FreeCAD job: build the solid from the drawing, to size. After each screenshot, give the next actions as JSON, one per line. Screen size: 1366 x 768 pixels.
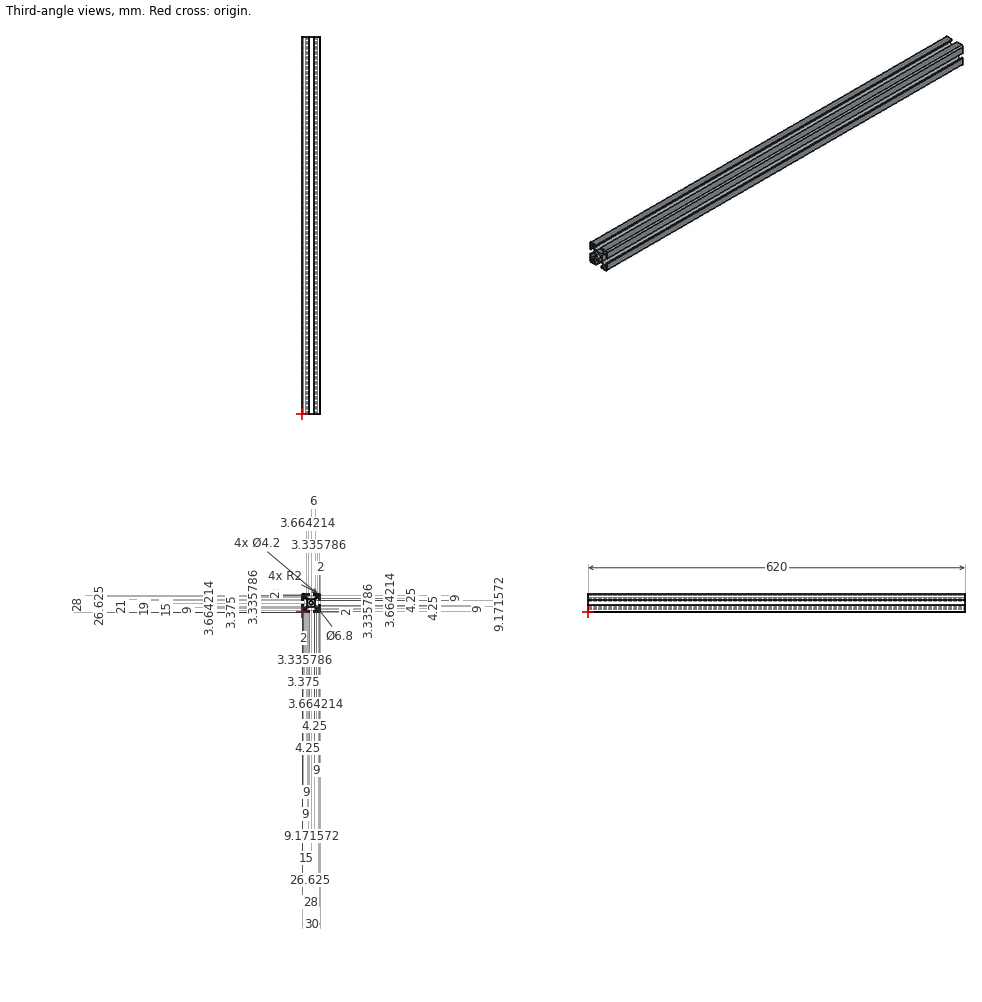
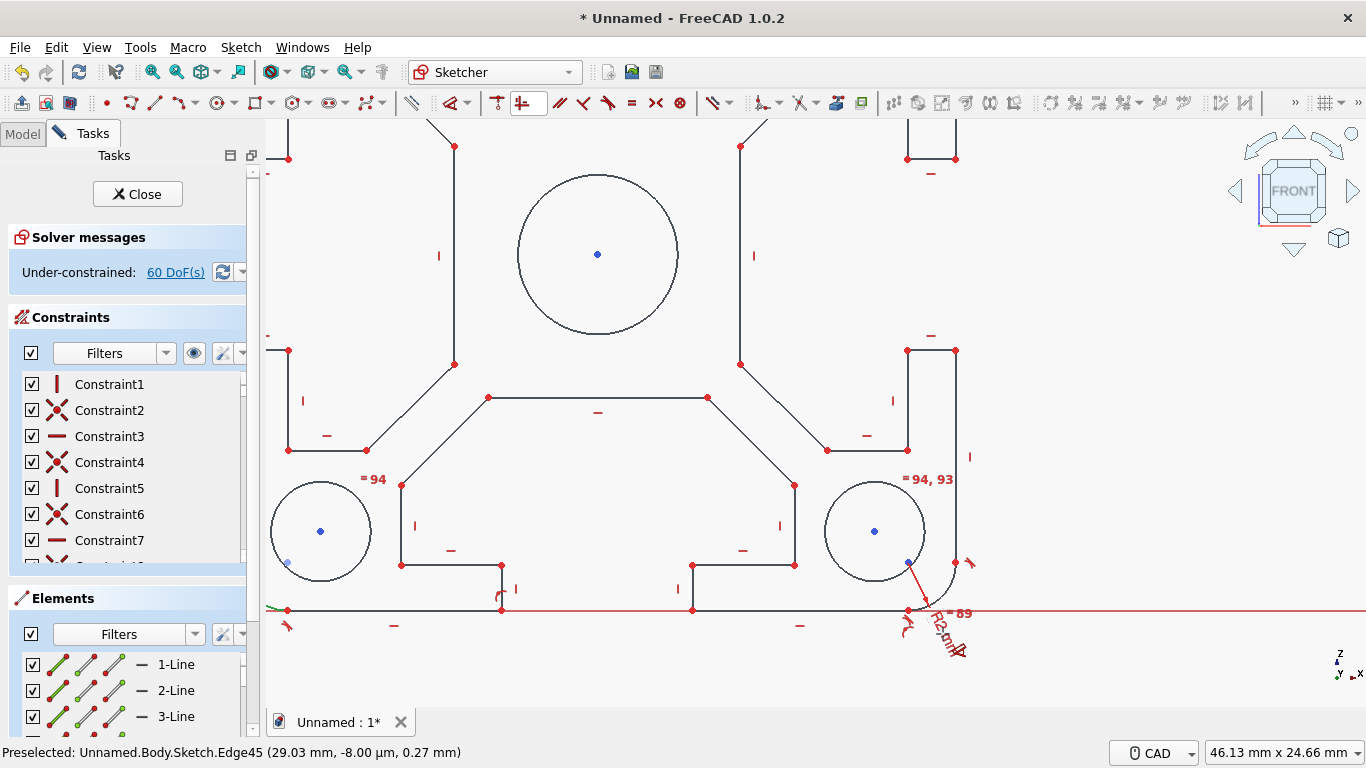
{"action": "scroll", "coordinate": [930, 608], "scroll_direction": "down", "scroll_amount": 3}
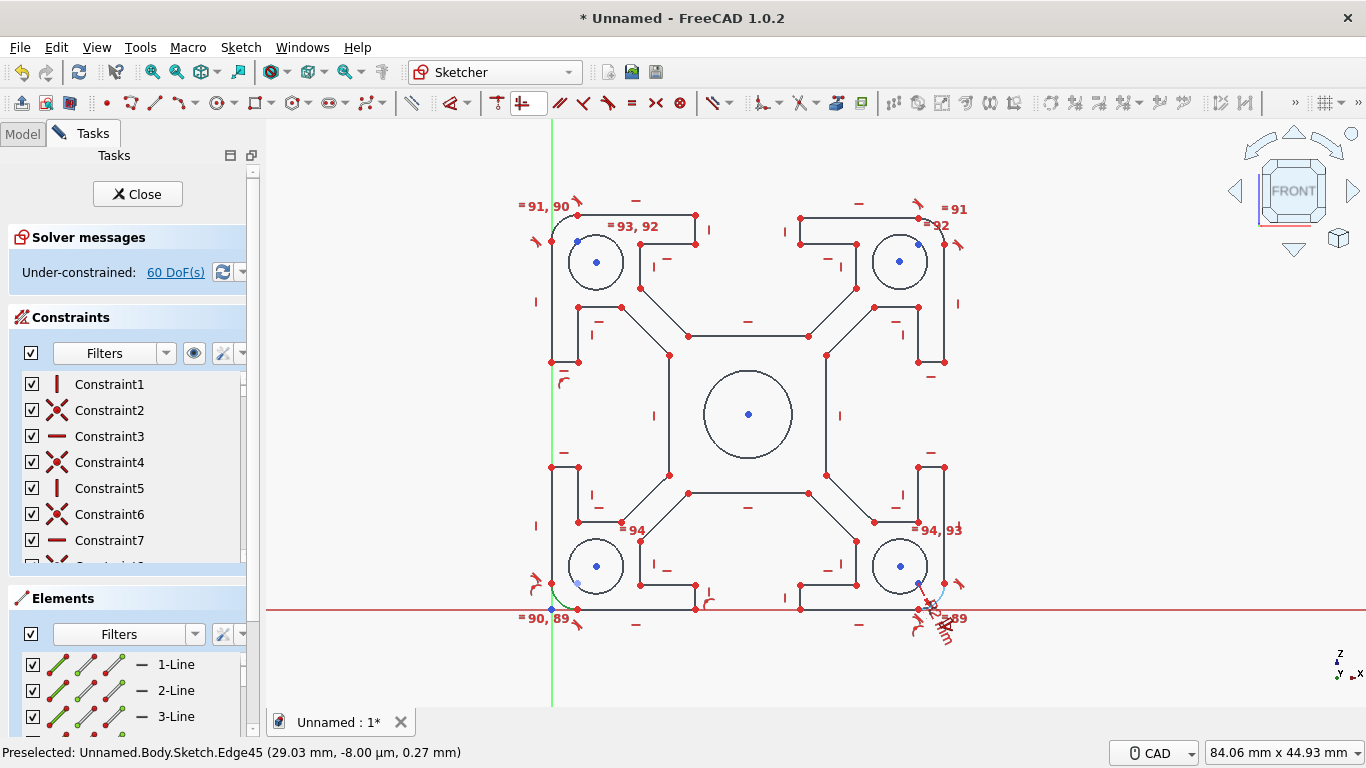
{"action": "left_click", "coordinate": [881, 243]}
{"action": "left_click", "coordinate": [912, 204]}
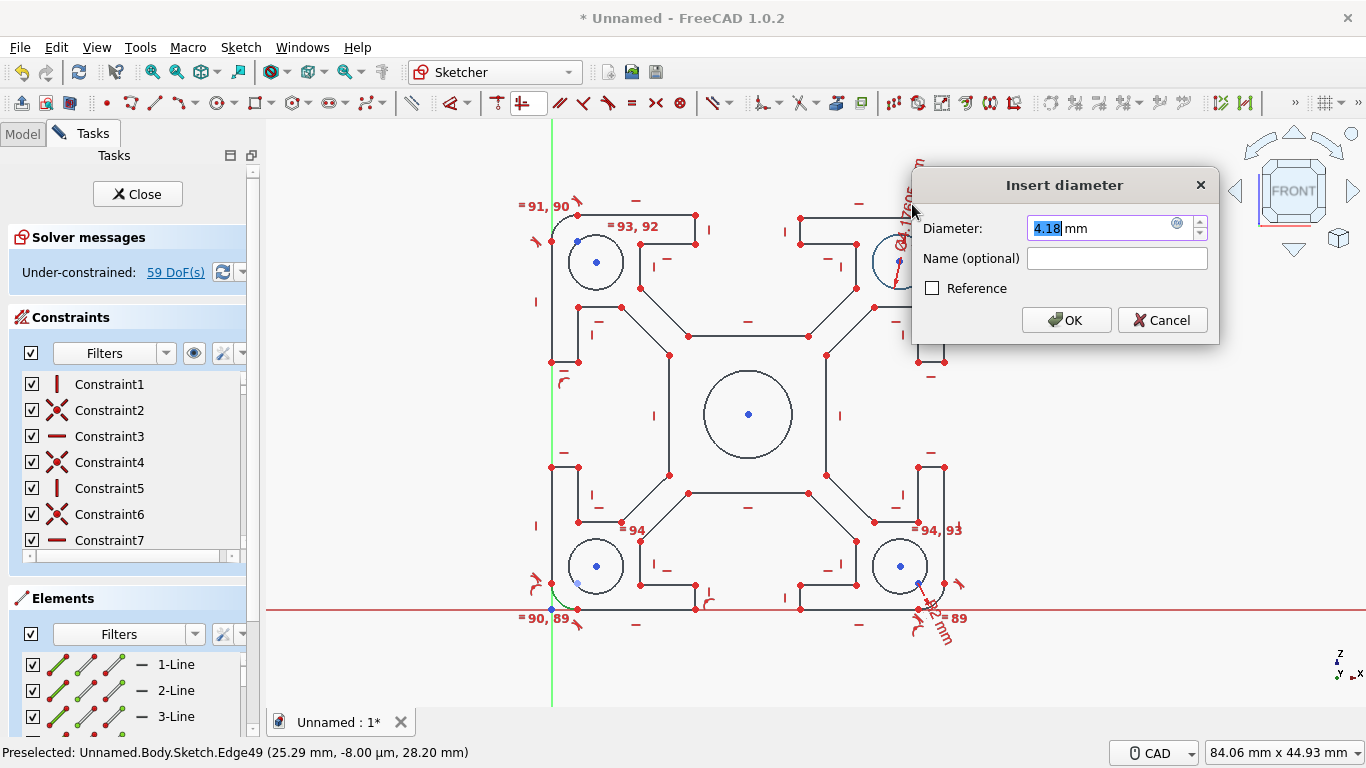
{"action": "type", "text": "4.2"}
{"action": "key", "text": "Return"}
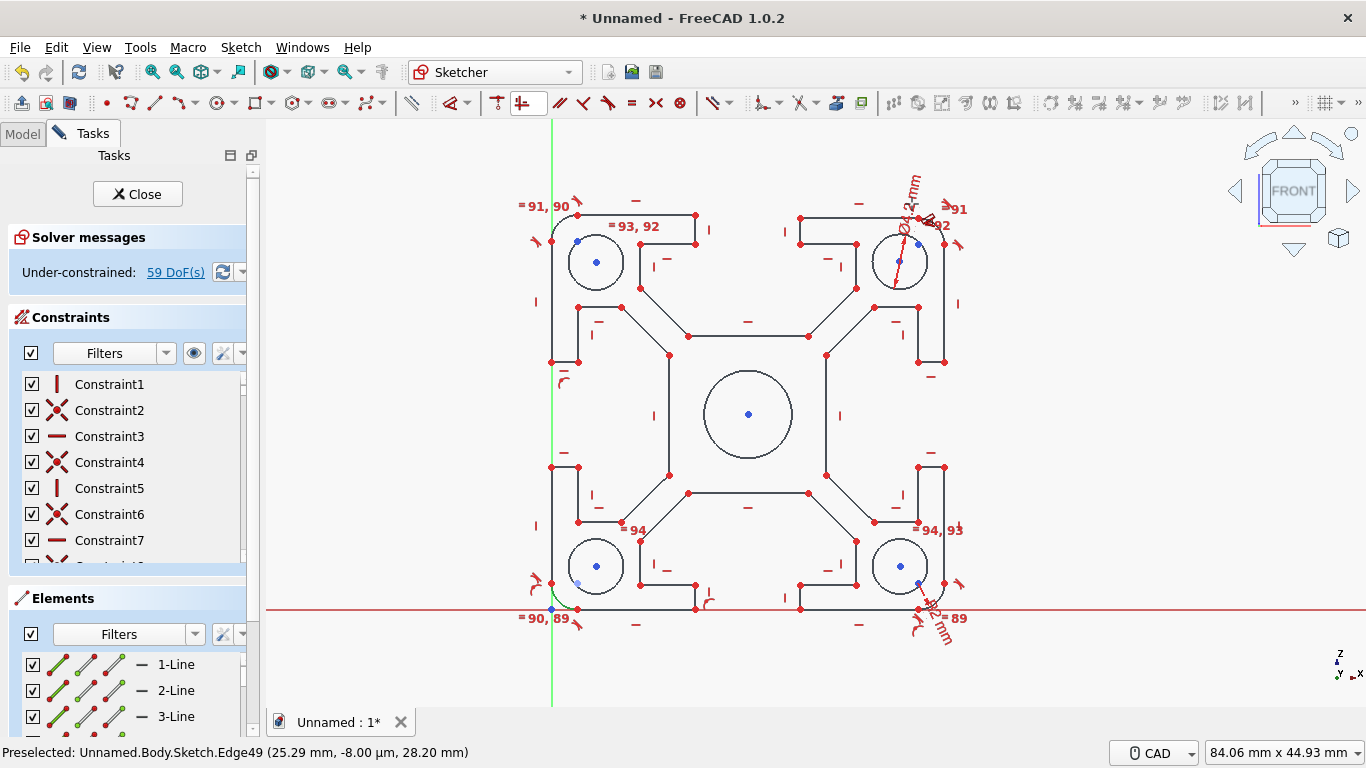
{"action": "left_click", "coordinate": [779, 383]}
{"action": "left_click", "coordinate": [801, 360]}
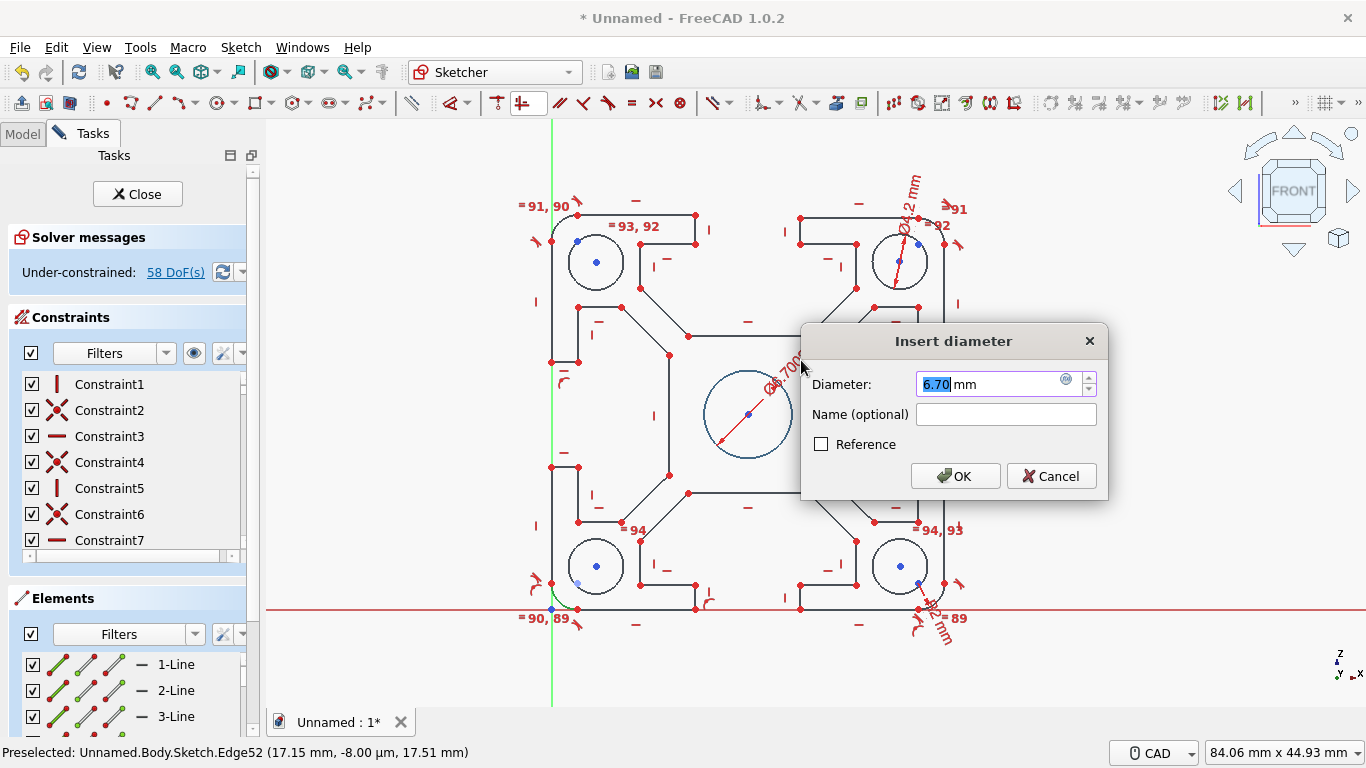
{"action": "type", "text": "6.8"}
{"action": "key", "text": "Return"}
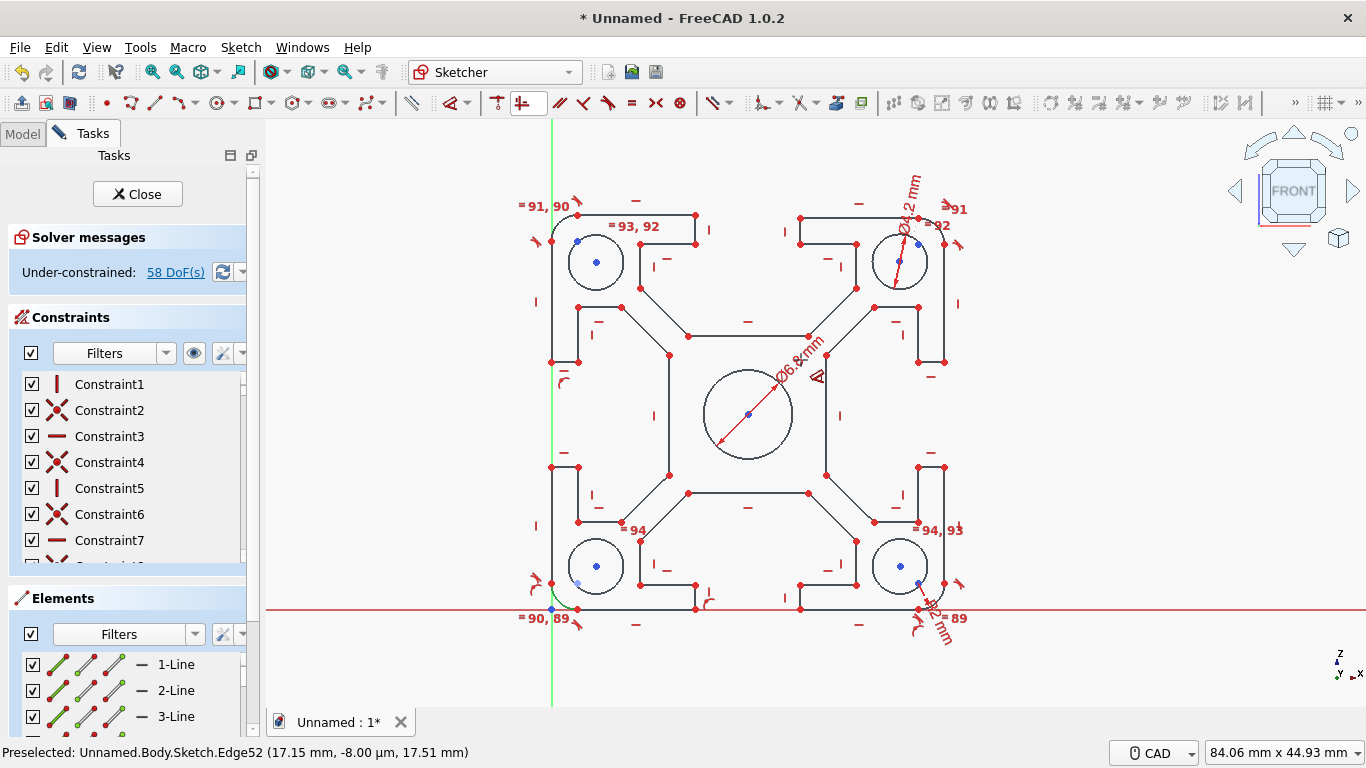
{"action": "left_click", "coordinate": [944, 280]}
{"action": "left_click", "coordinate": [978, 303]}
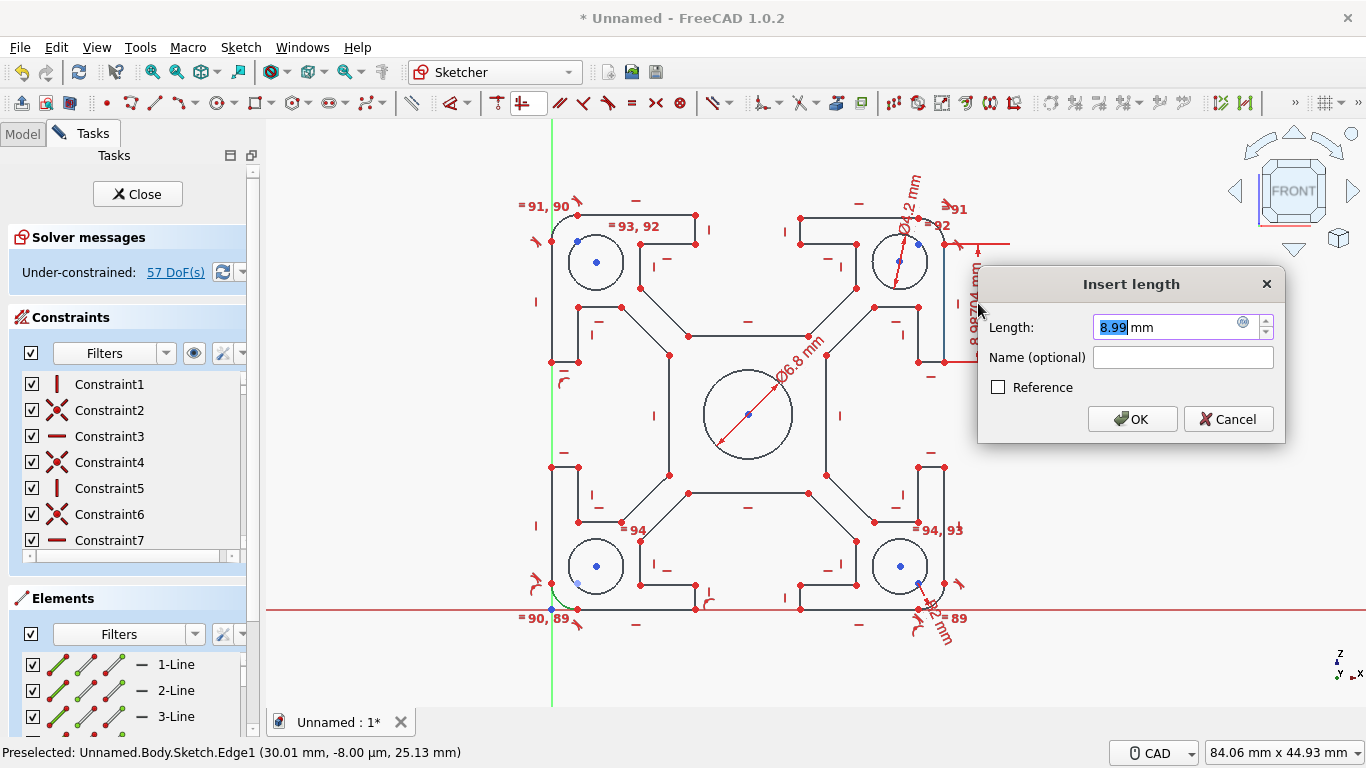
{"action": "type", "text": "9"}
{"action": "key", "text": "Return"}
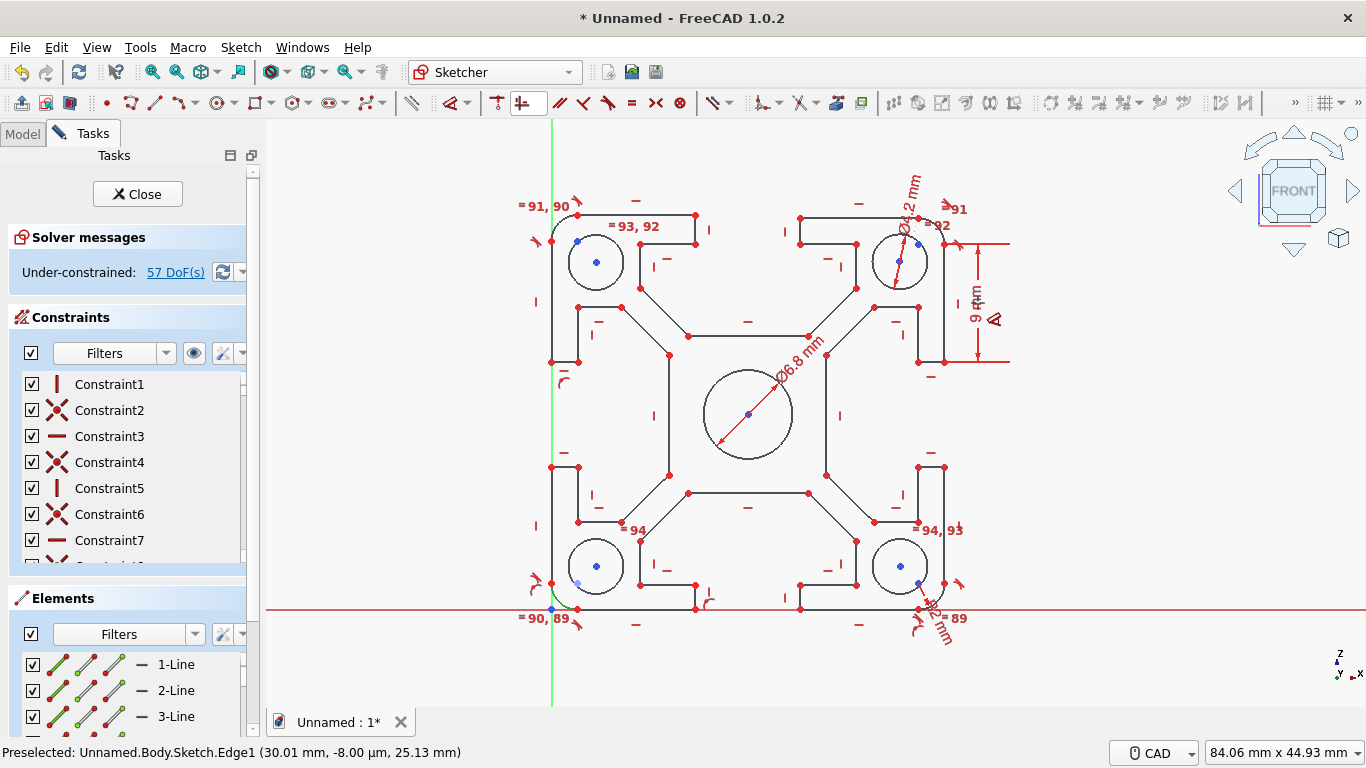
{"action": "scroll", "coordinate": [934, 362], "scroll_direction": "up", "scroll_amount": 3}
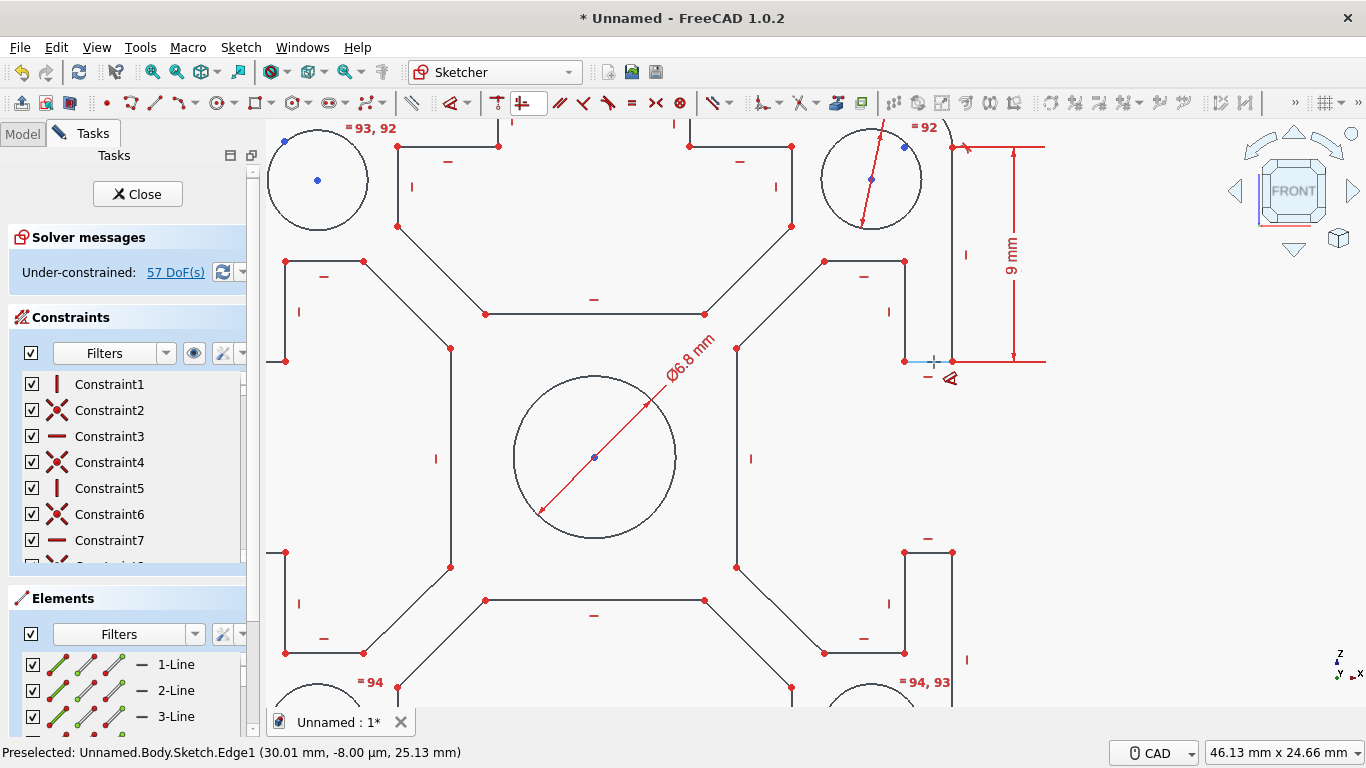
{"action": "left_click", "coordinate": [933, 362]}
{"action": "left_click", "coordinate": [928, 328]}